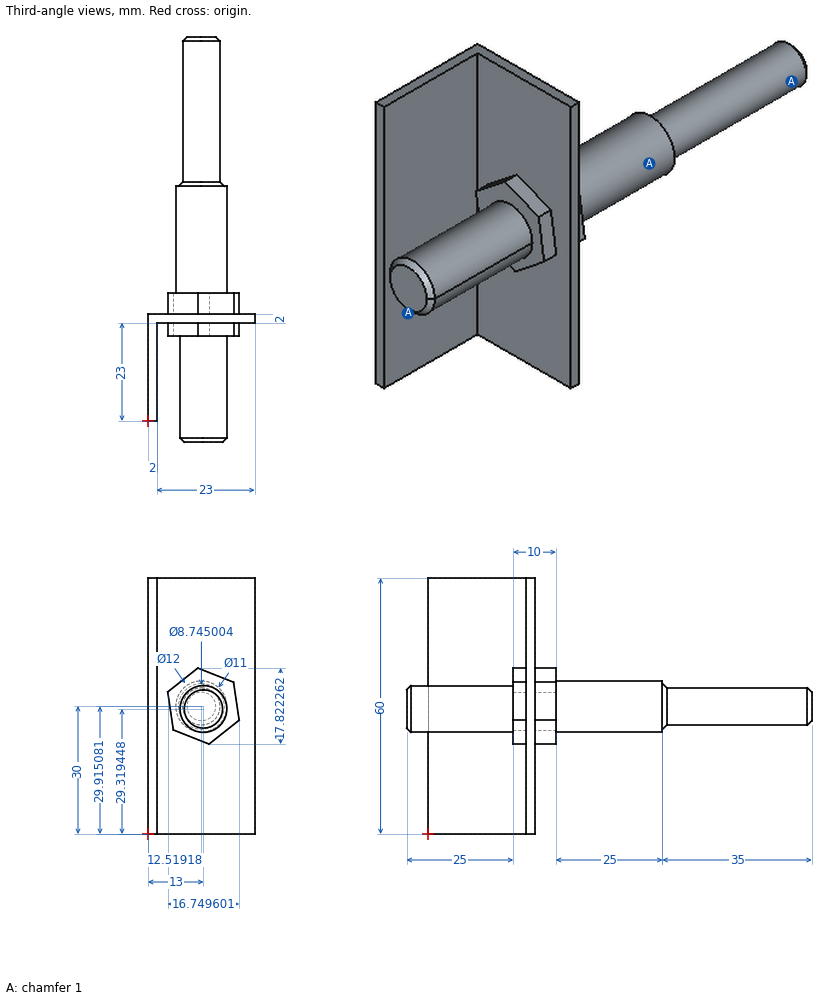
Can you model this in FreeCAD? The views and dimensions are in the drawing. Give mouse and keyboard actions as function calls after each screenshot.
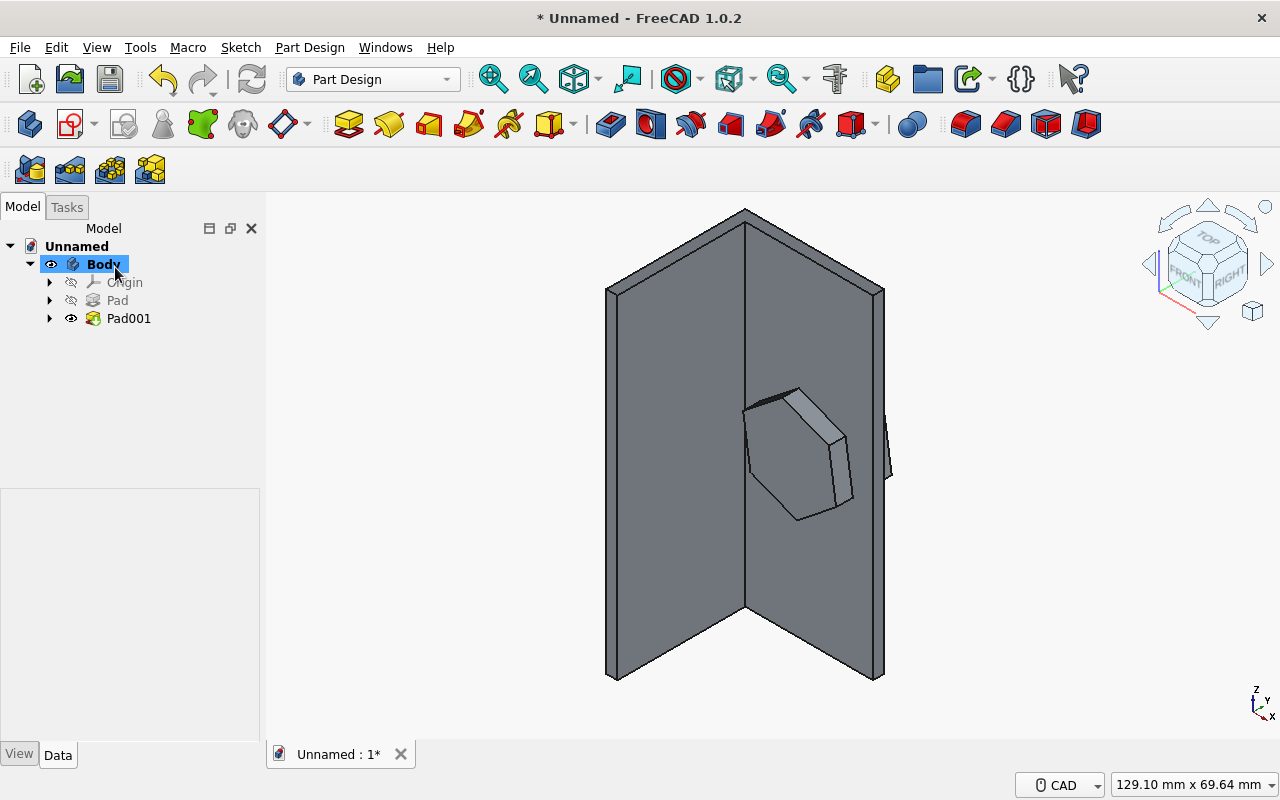
click(494, 80)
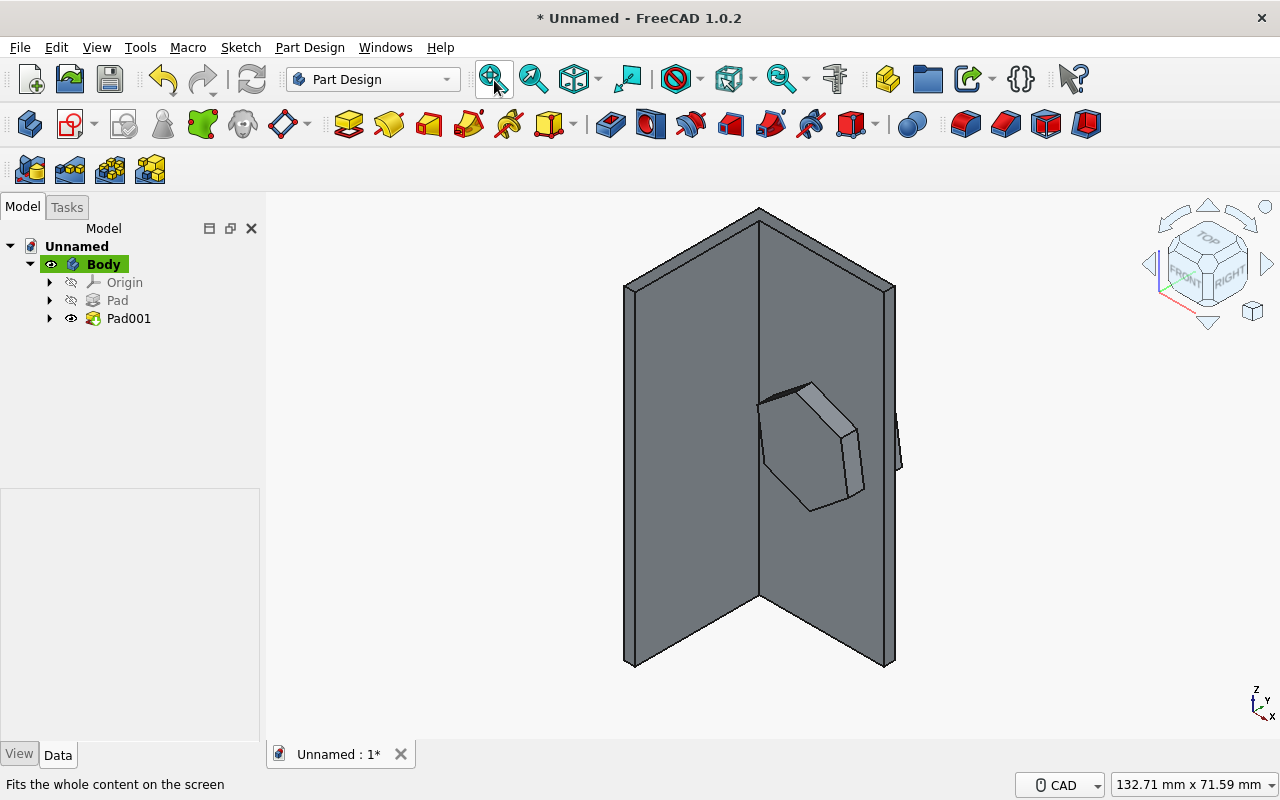
click(803, 450)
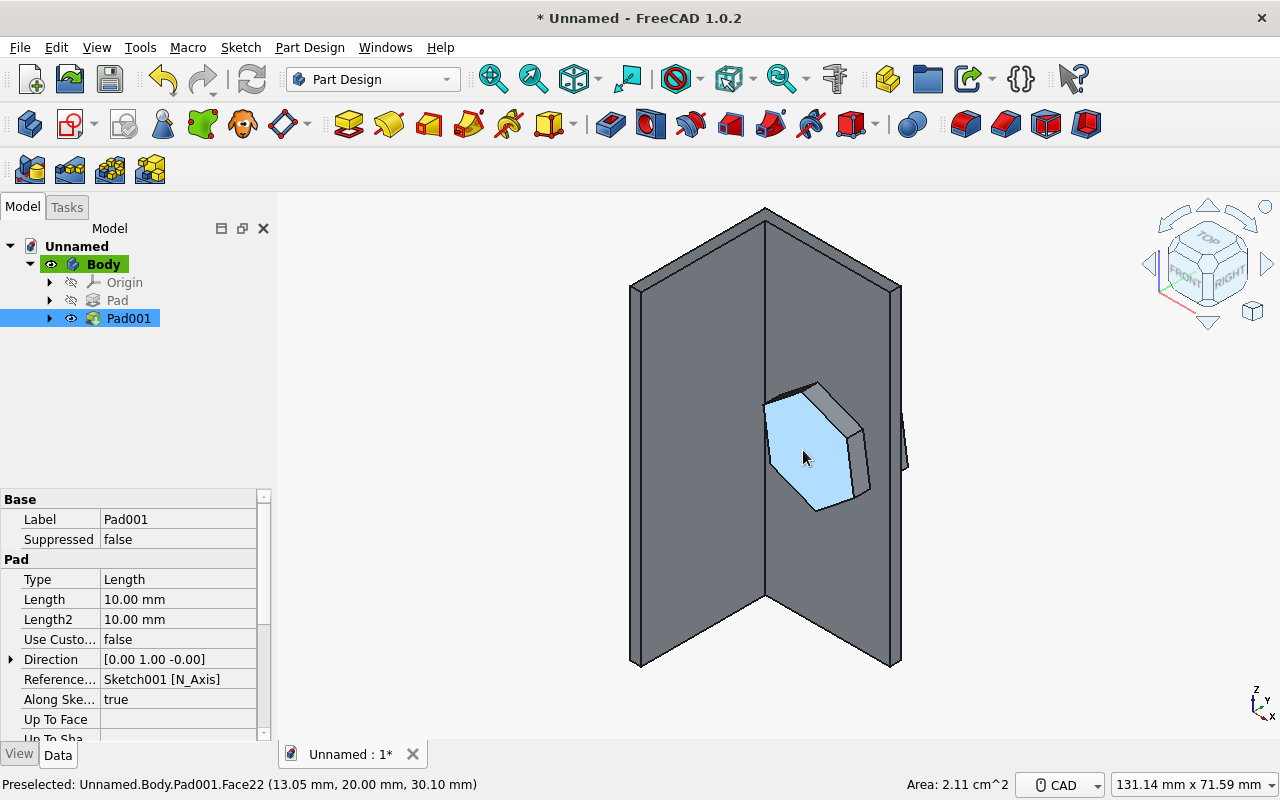
click(70, 124)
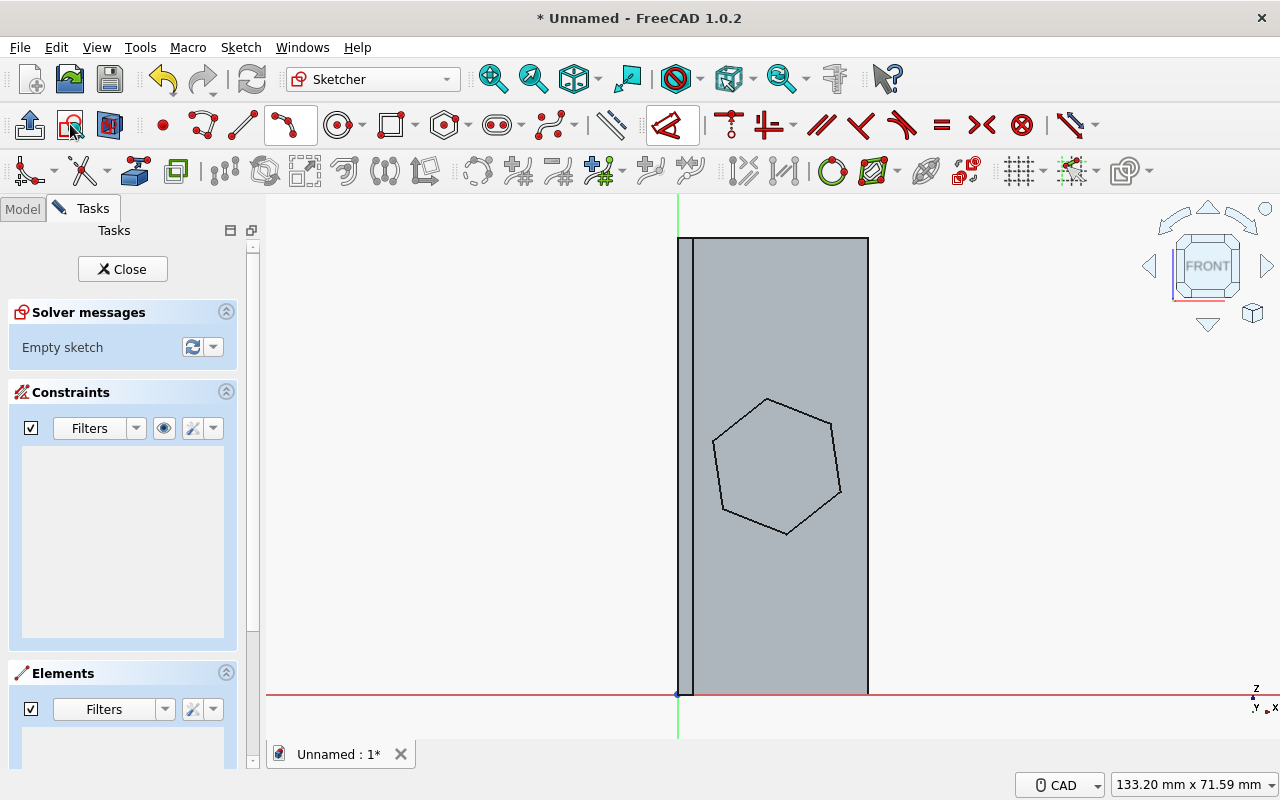
key(q)
key(s)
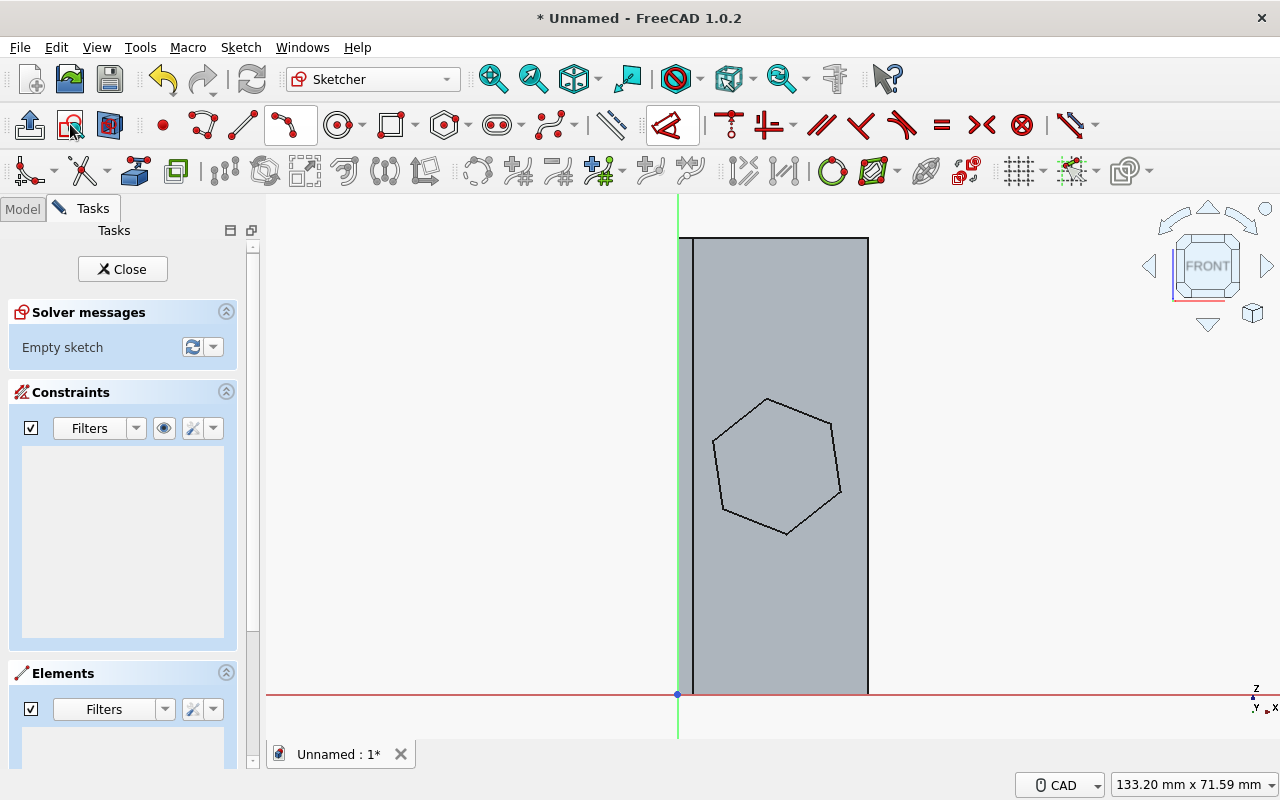
scroll(800, 473, up, 7)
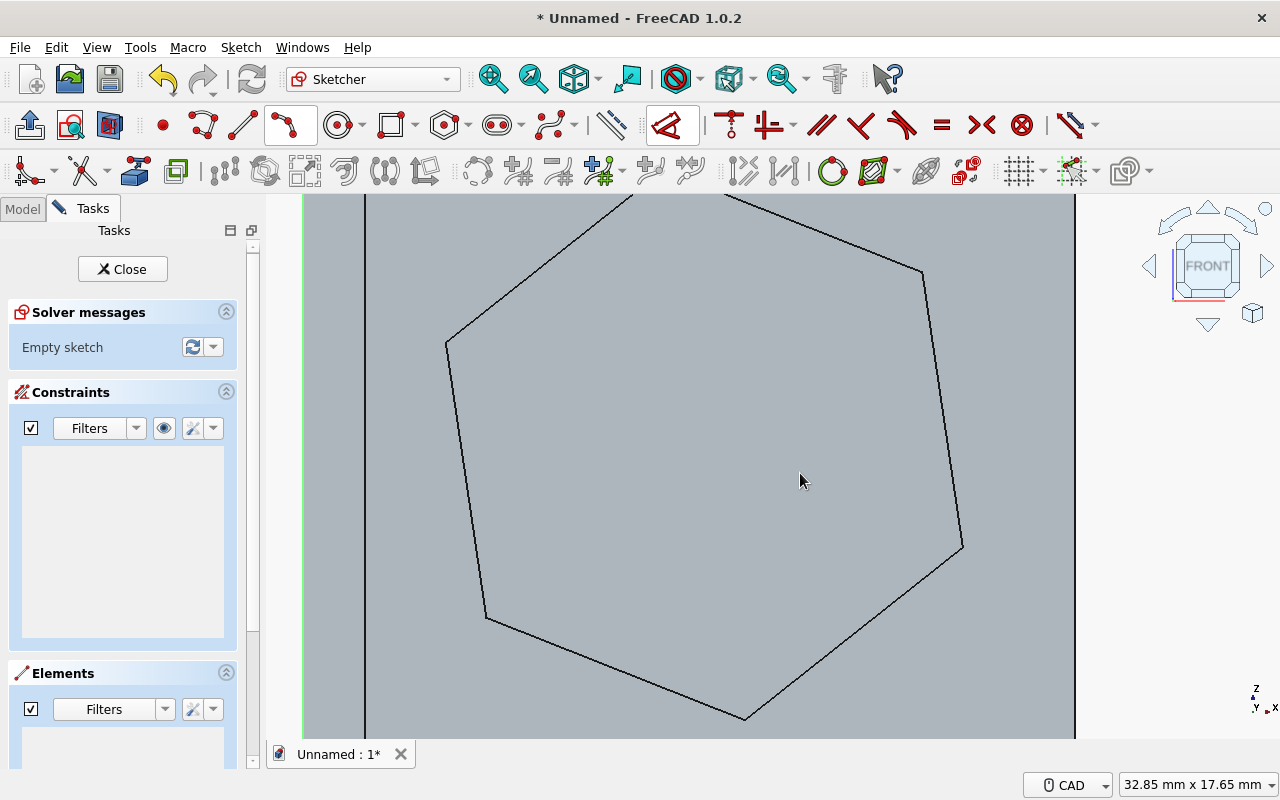
click(338, 126)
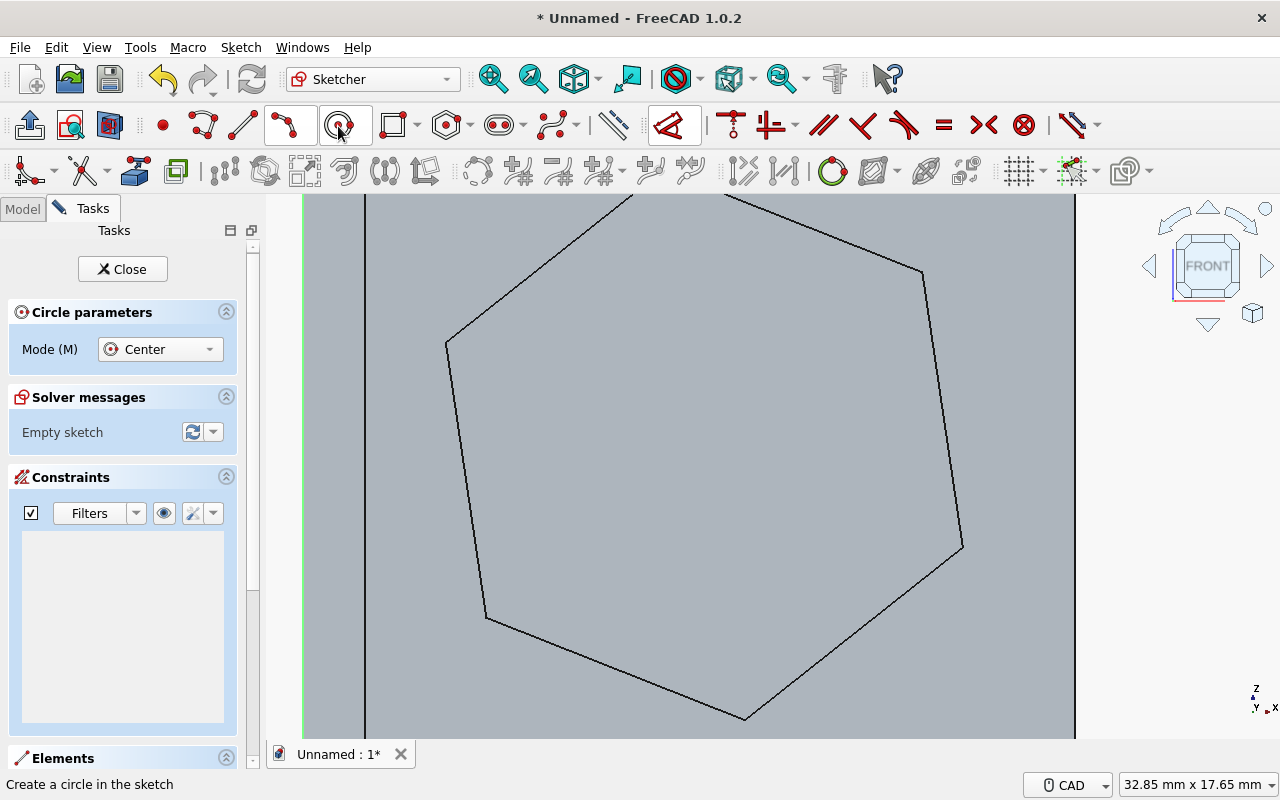
click(704, 466)
click(824, 346)
key(Escape)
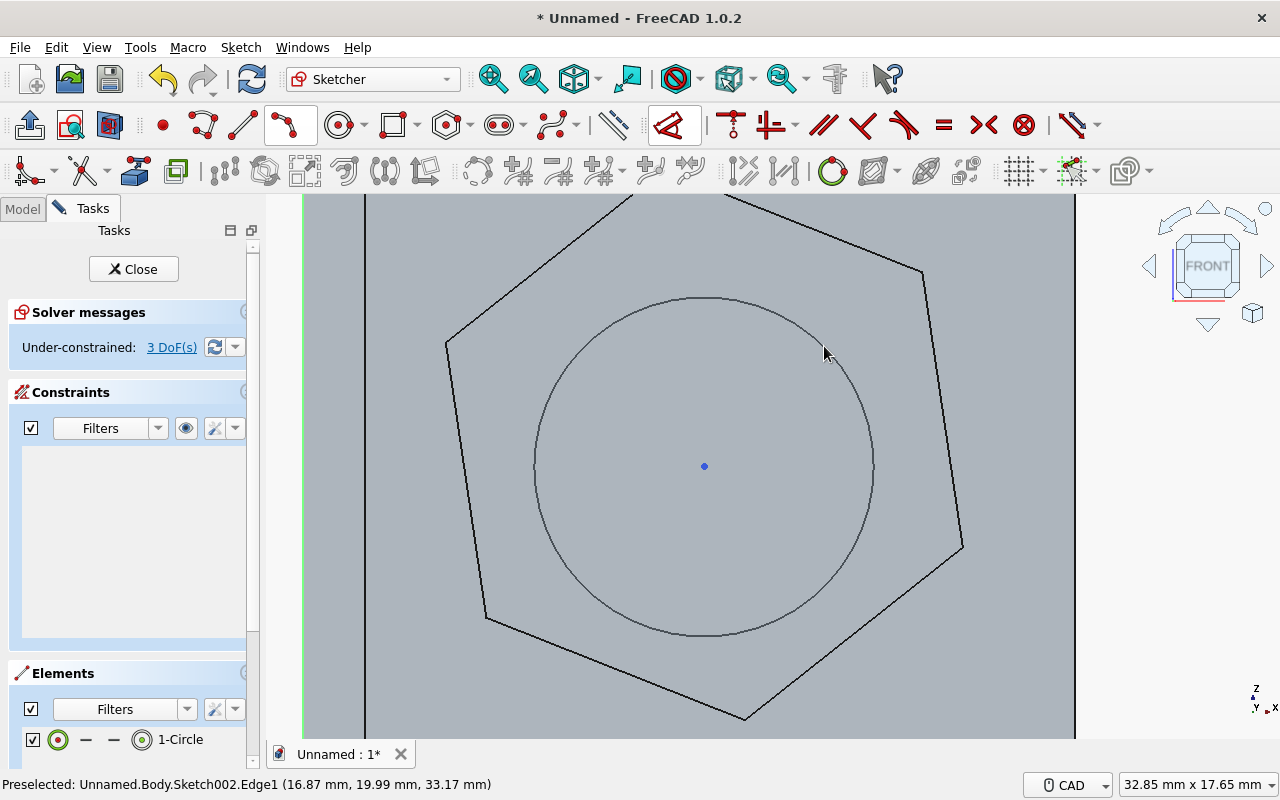
click(824, 347)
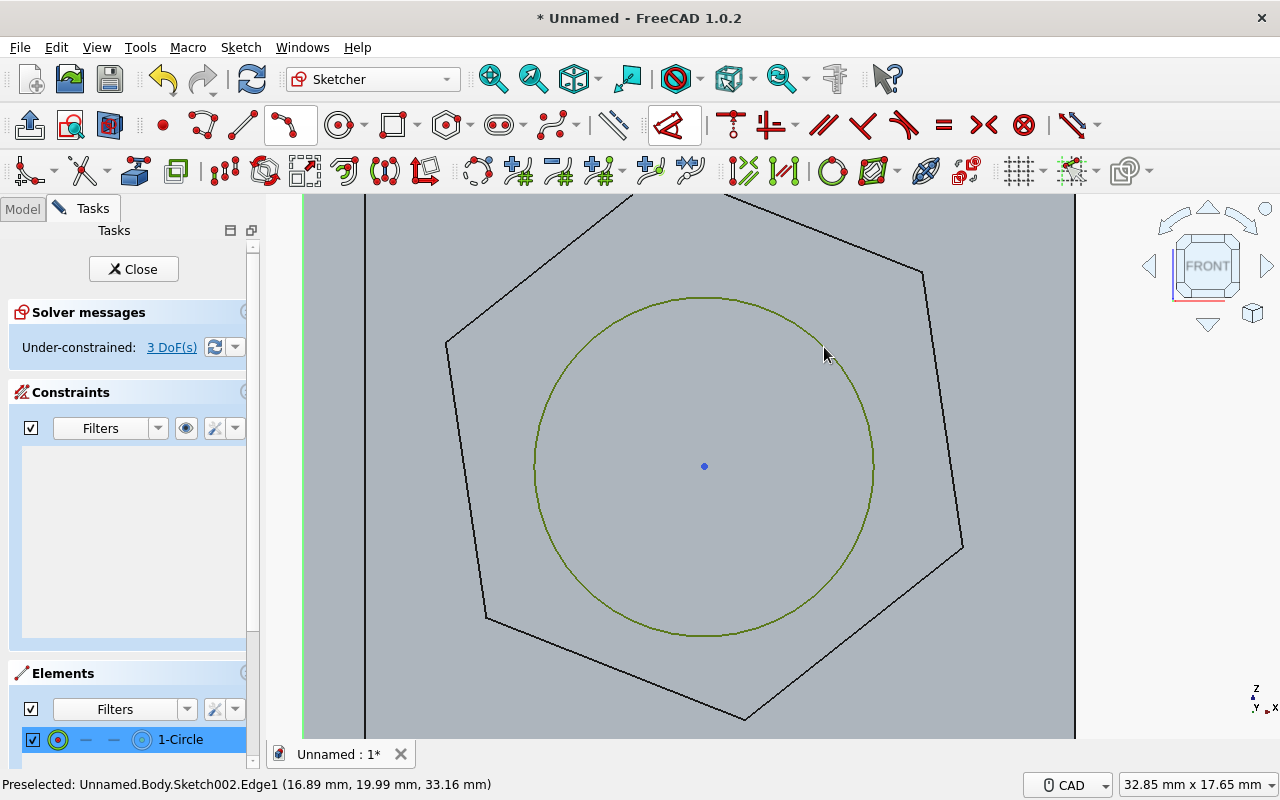
click(696, 126)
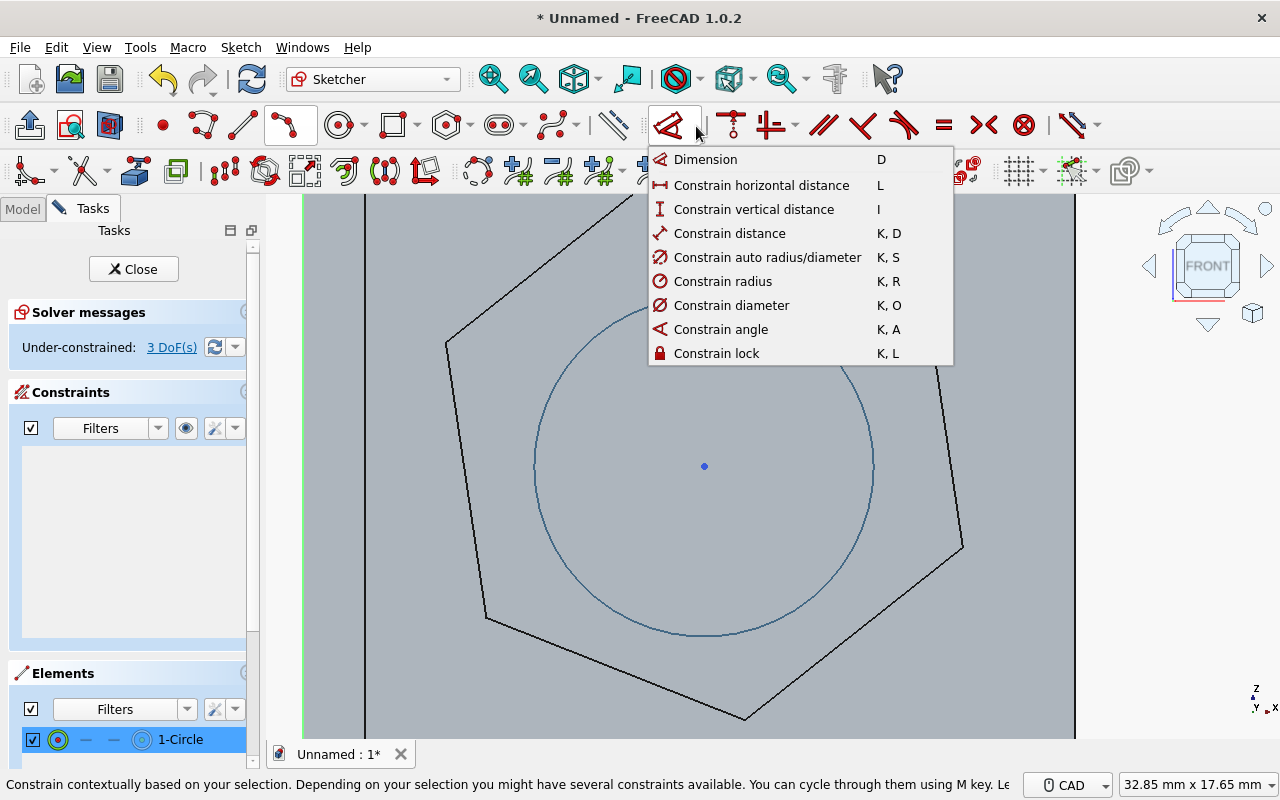
click(801, 305)